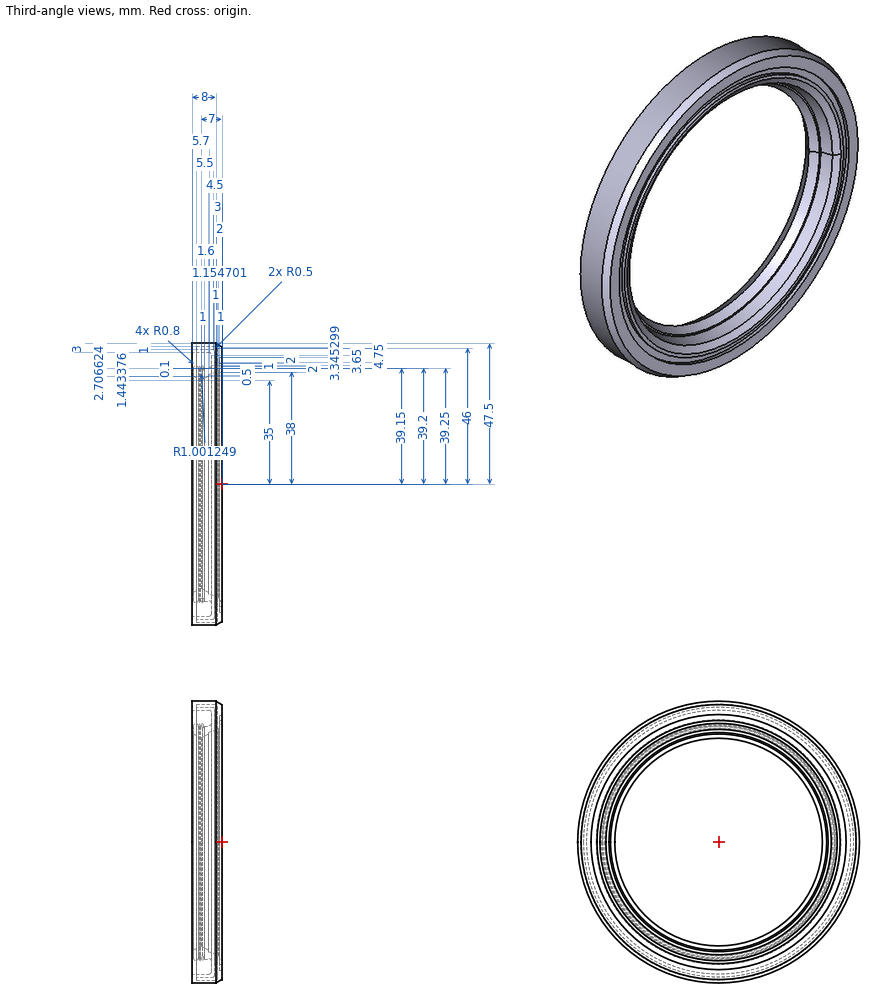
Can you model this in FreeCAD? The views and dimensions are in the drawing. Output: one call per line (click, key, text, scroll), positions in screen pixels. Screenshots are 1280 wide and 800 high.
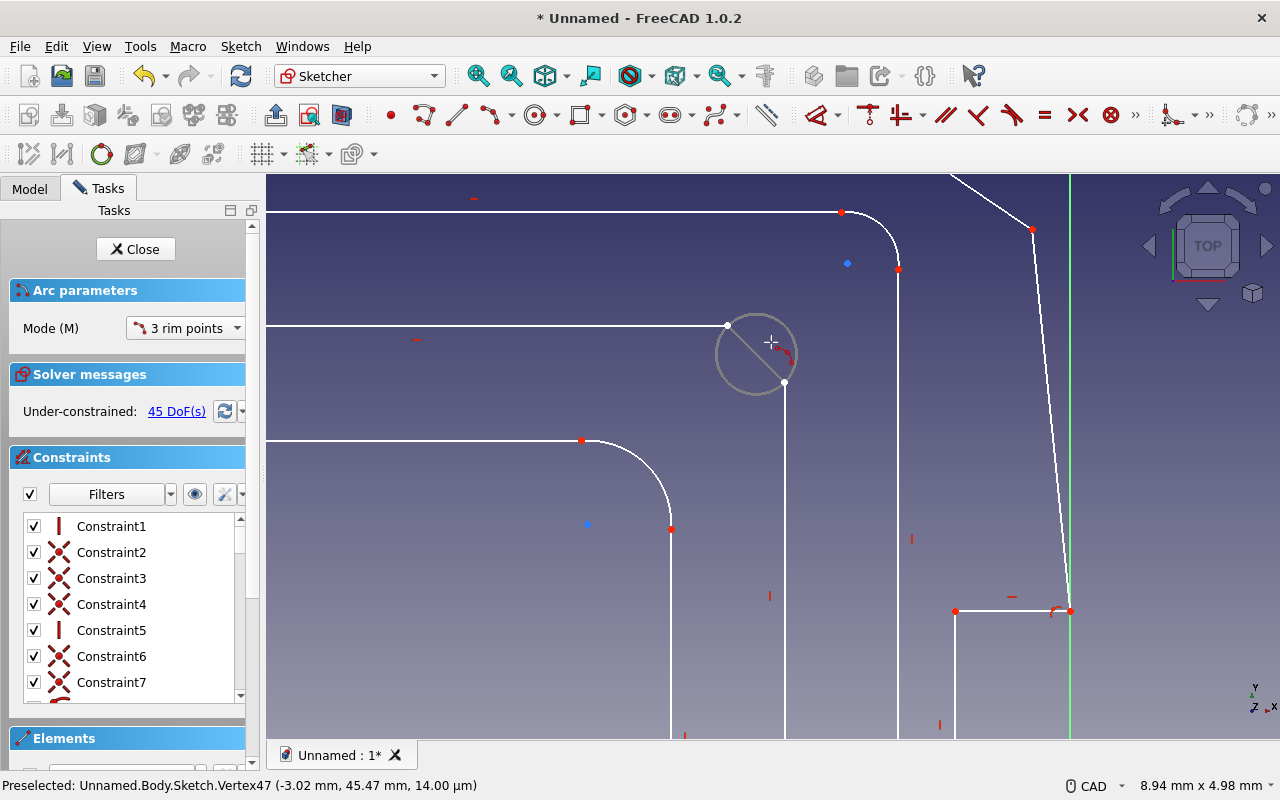
click(770, 339)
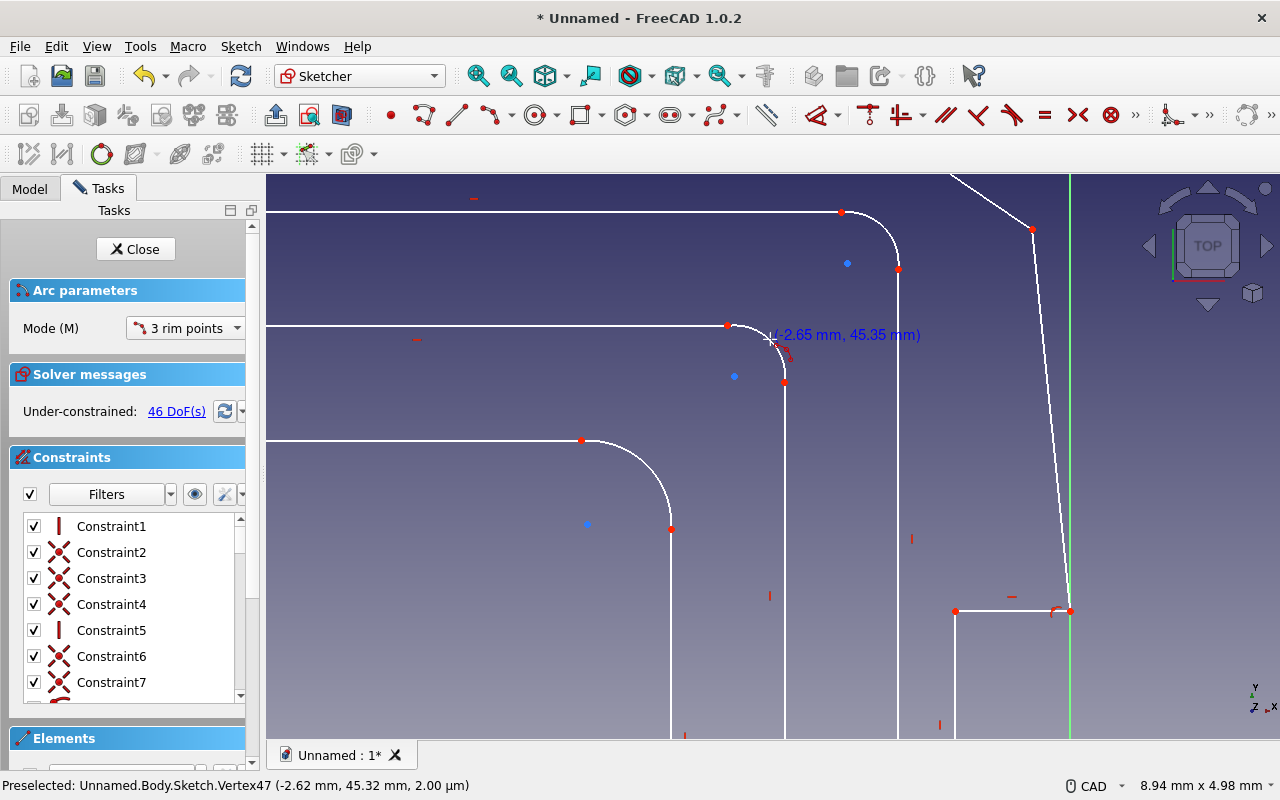
click(534, 116)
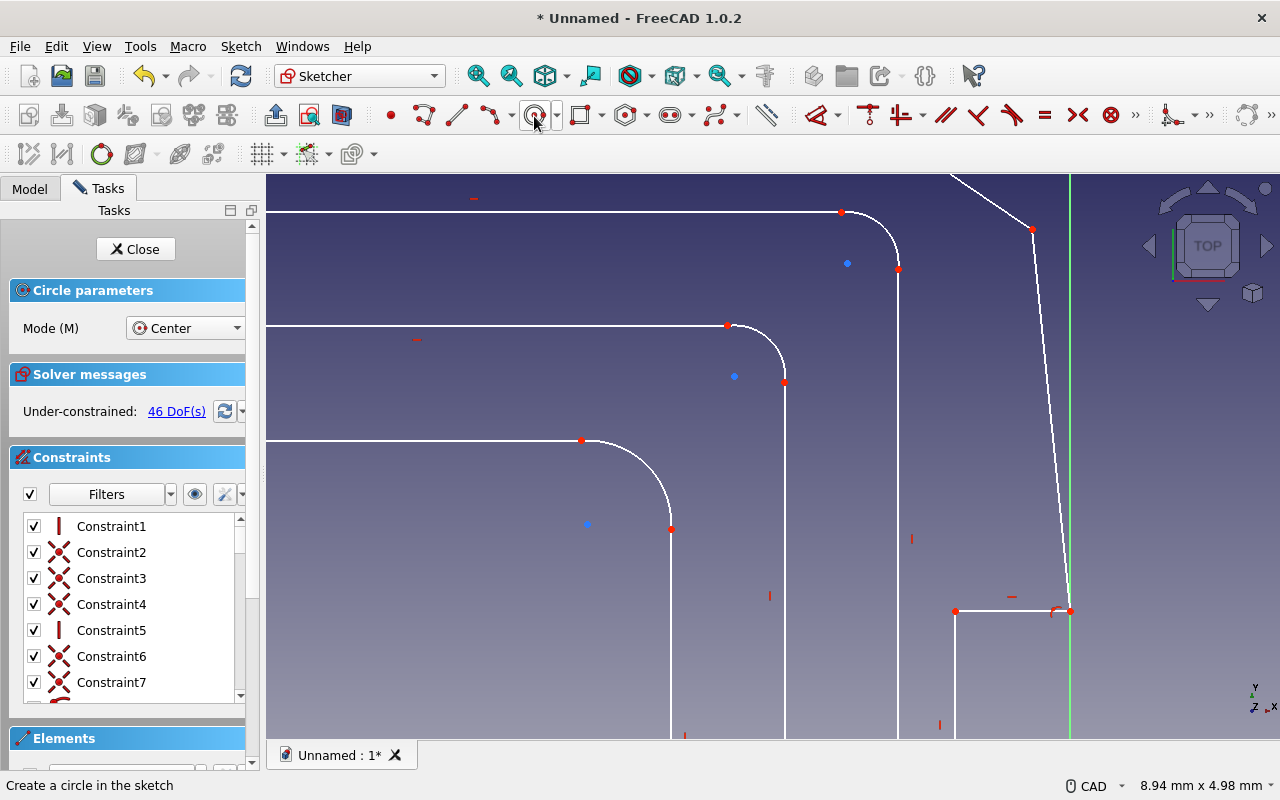
scroll(770, 342, down, 7)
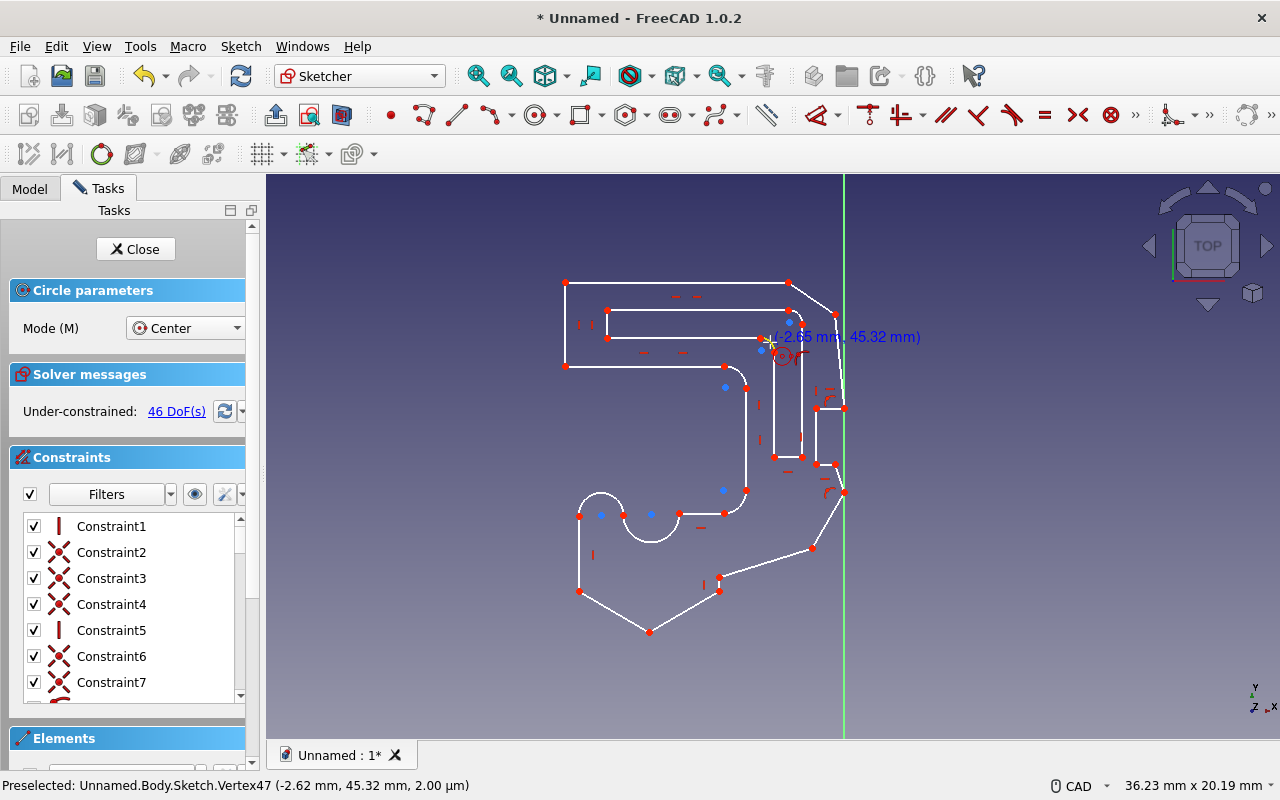
scroll(651, 512, up, 13)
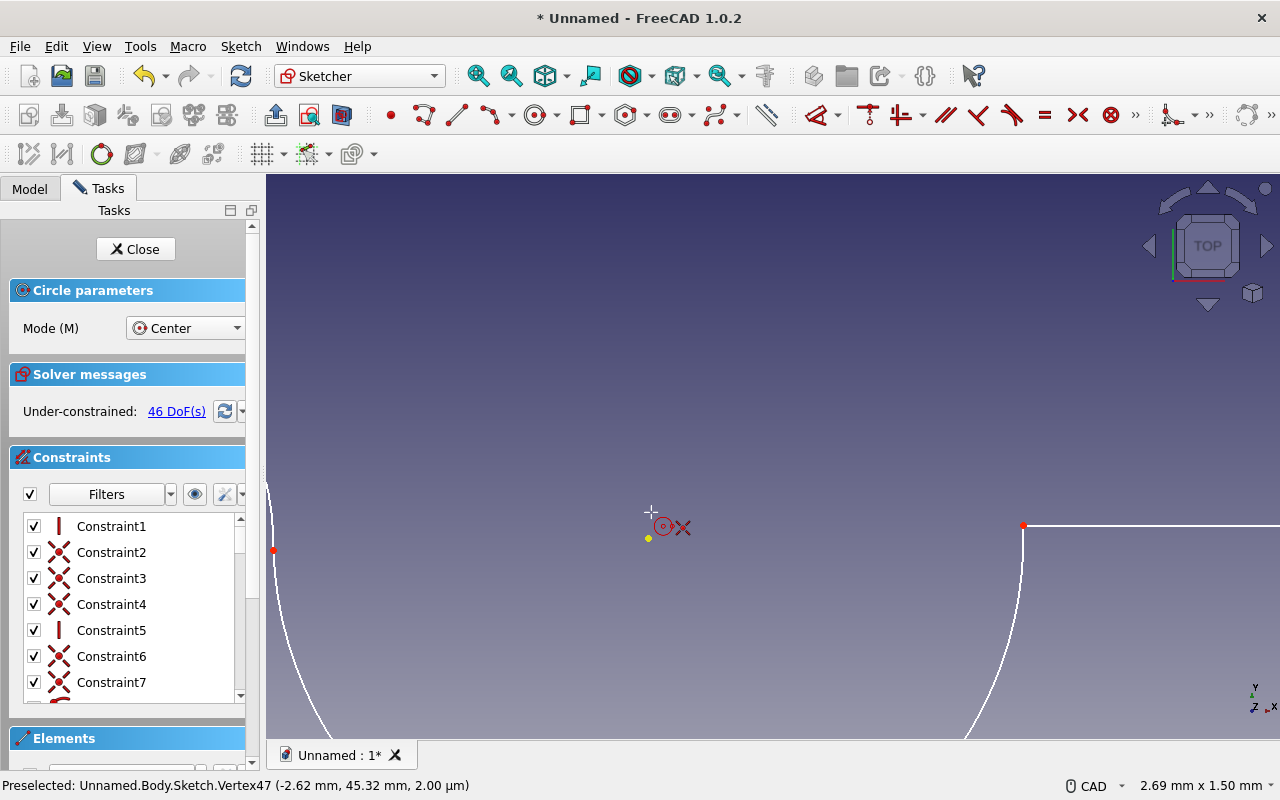
click(651, 510)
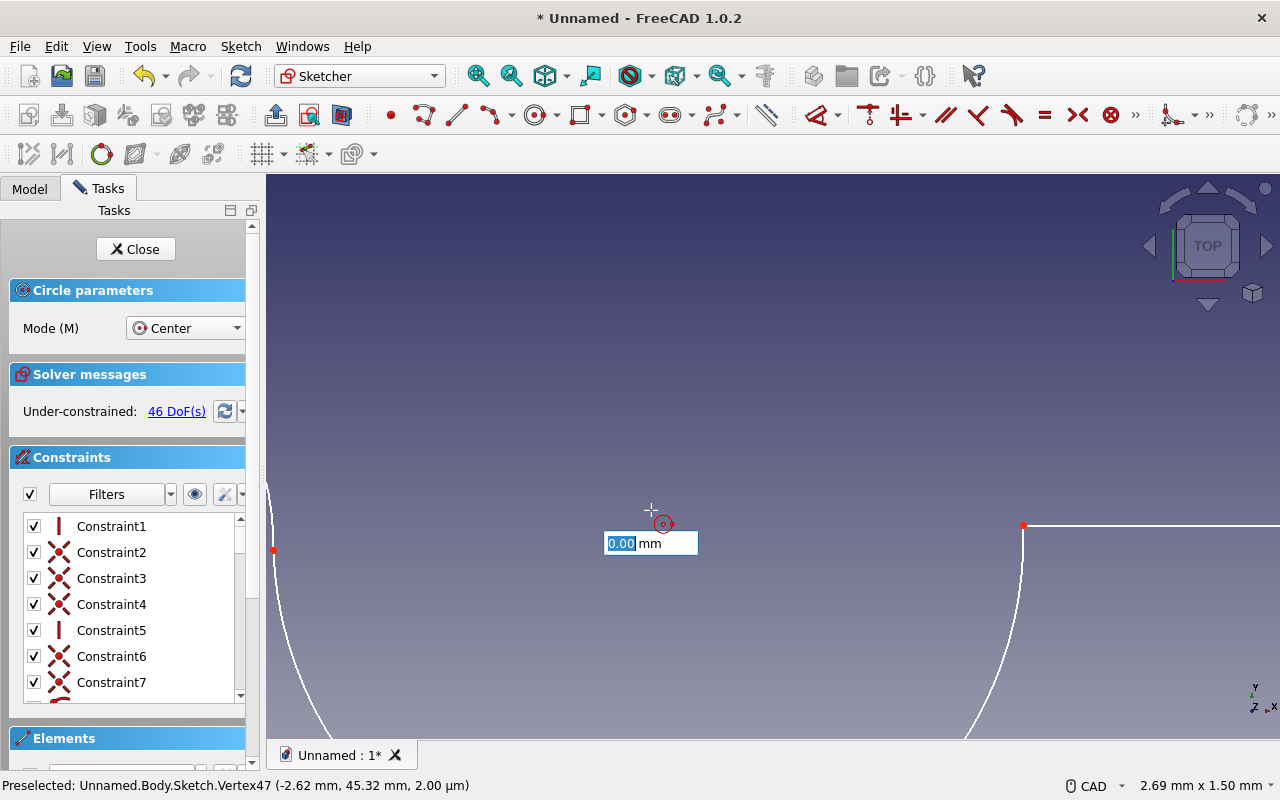
scroll(651, 513, down, 13)
move(667, 497)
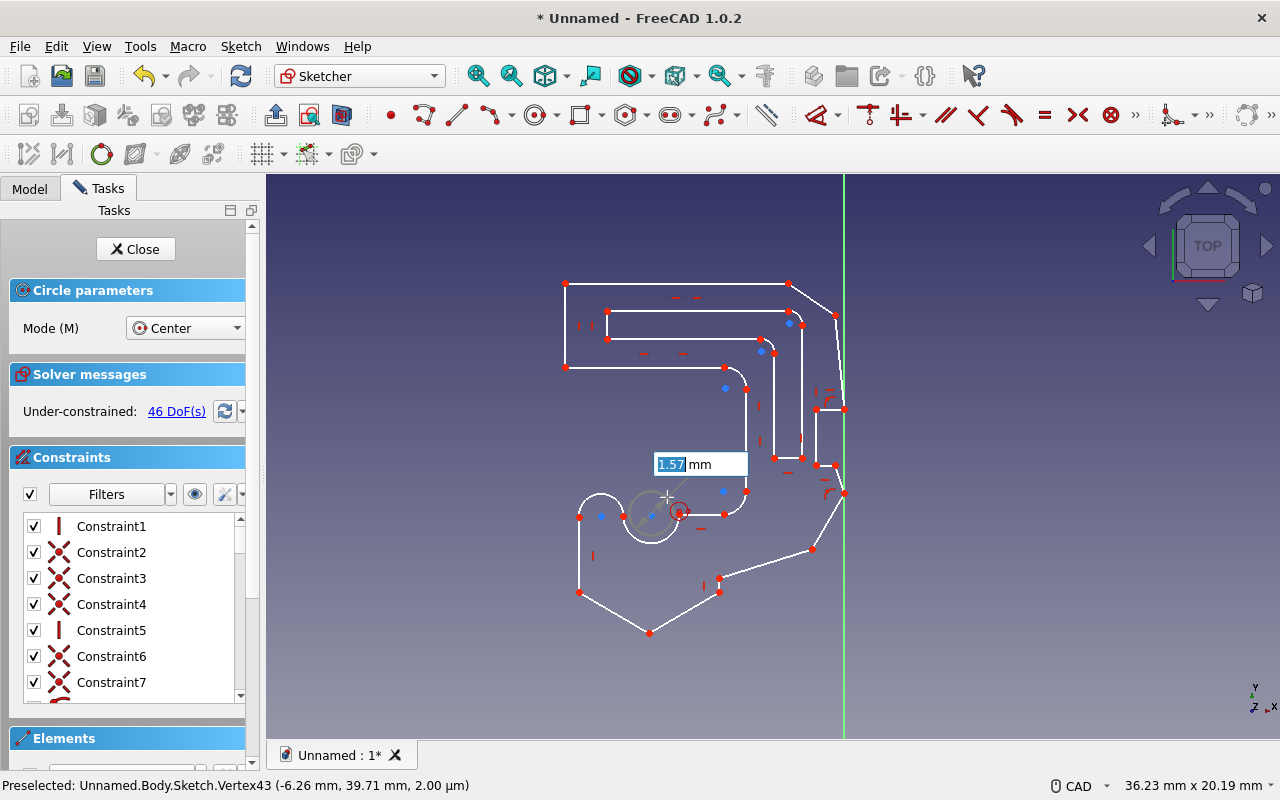
text(1.6)
key(Return)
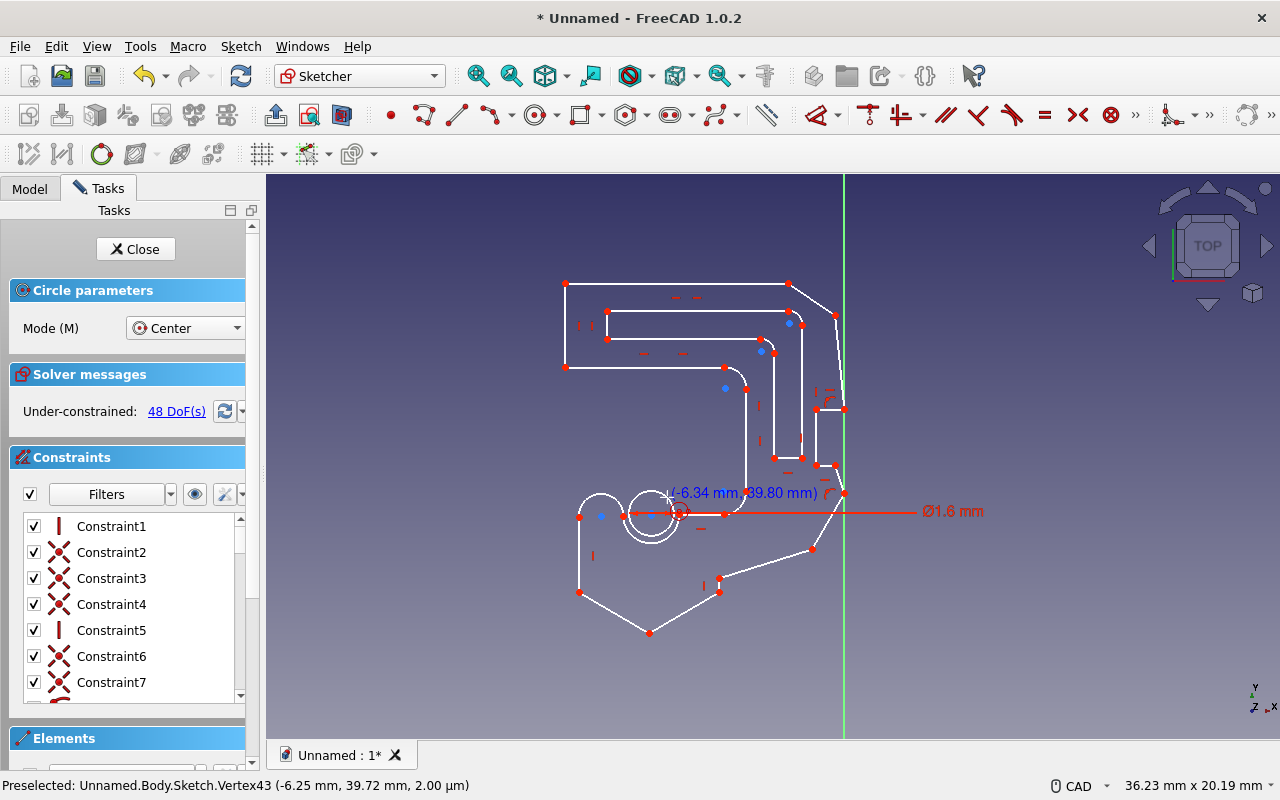
scroll(651, 513, up, 13)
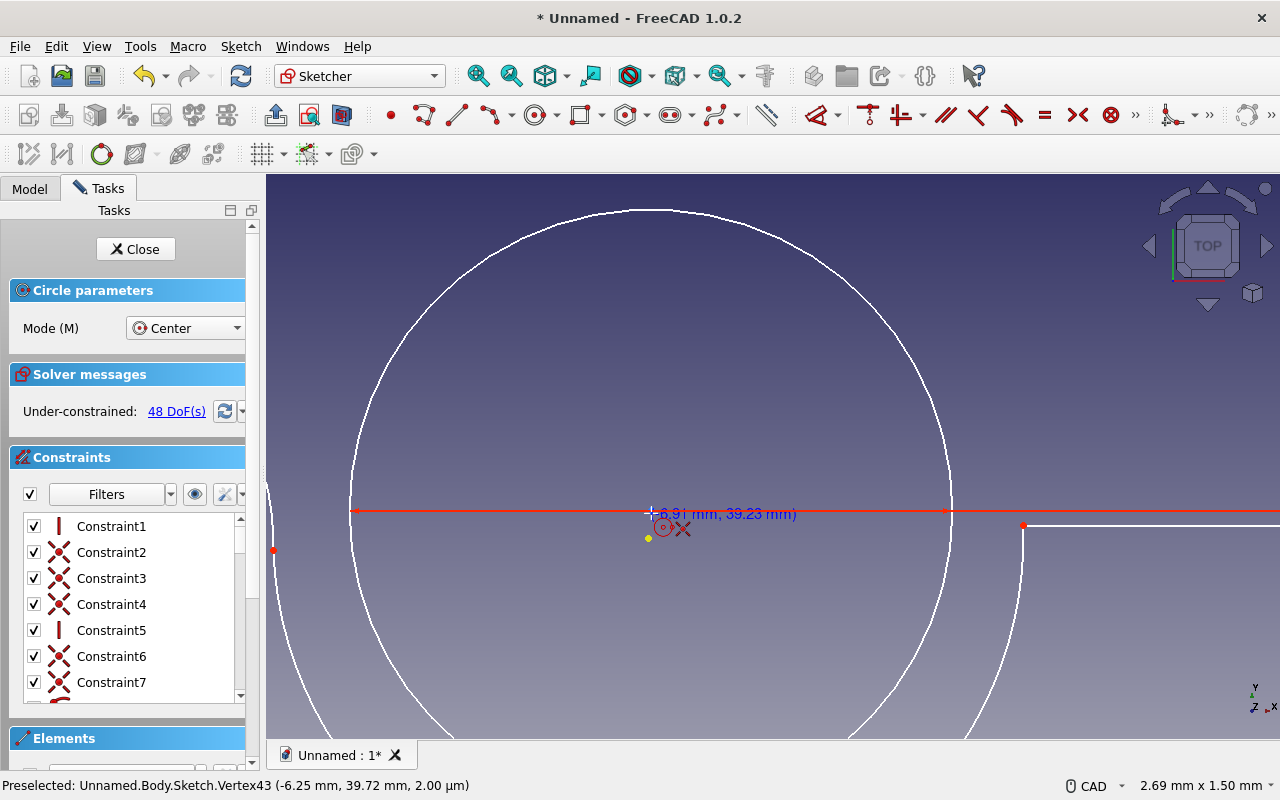
click(651, 511)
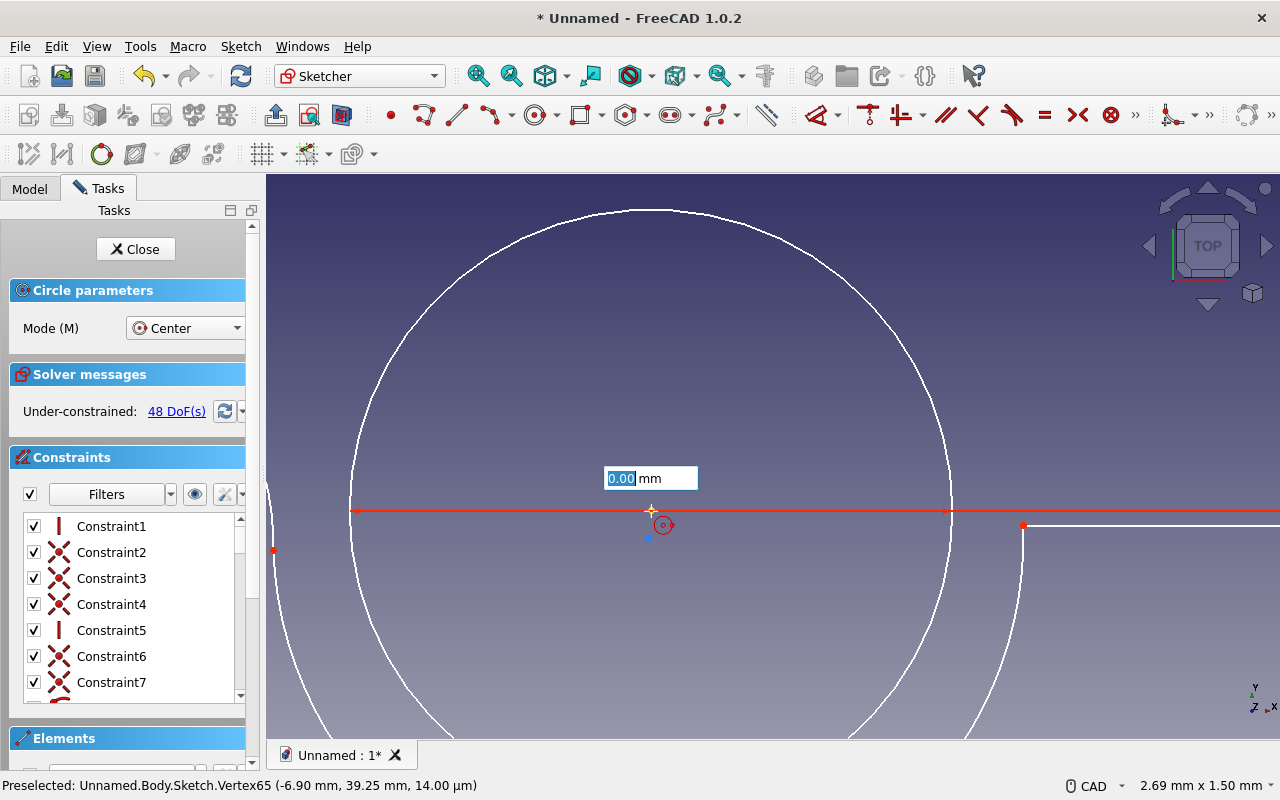
scroll(651, 513, down, 13)